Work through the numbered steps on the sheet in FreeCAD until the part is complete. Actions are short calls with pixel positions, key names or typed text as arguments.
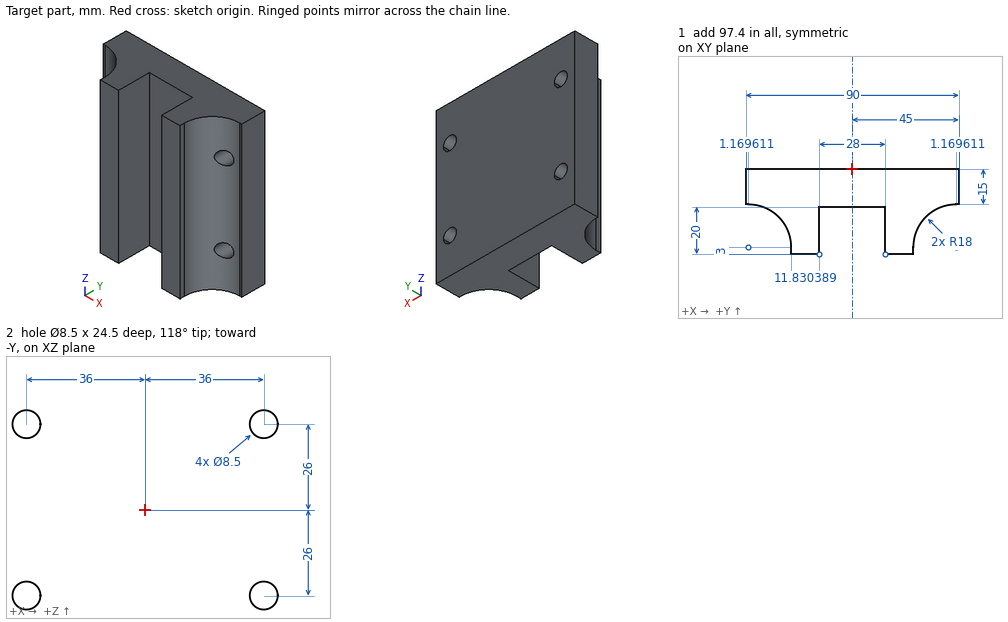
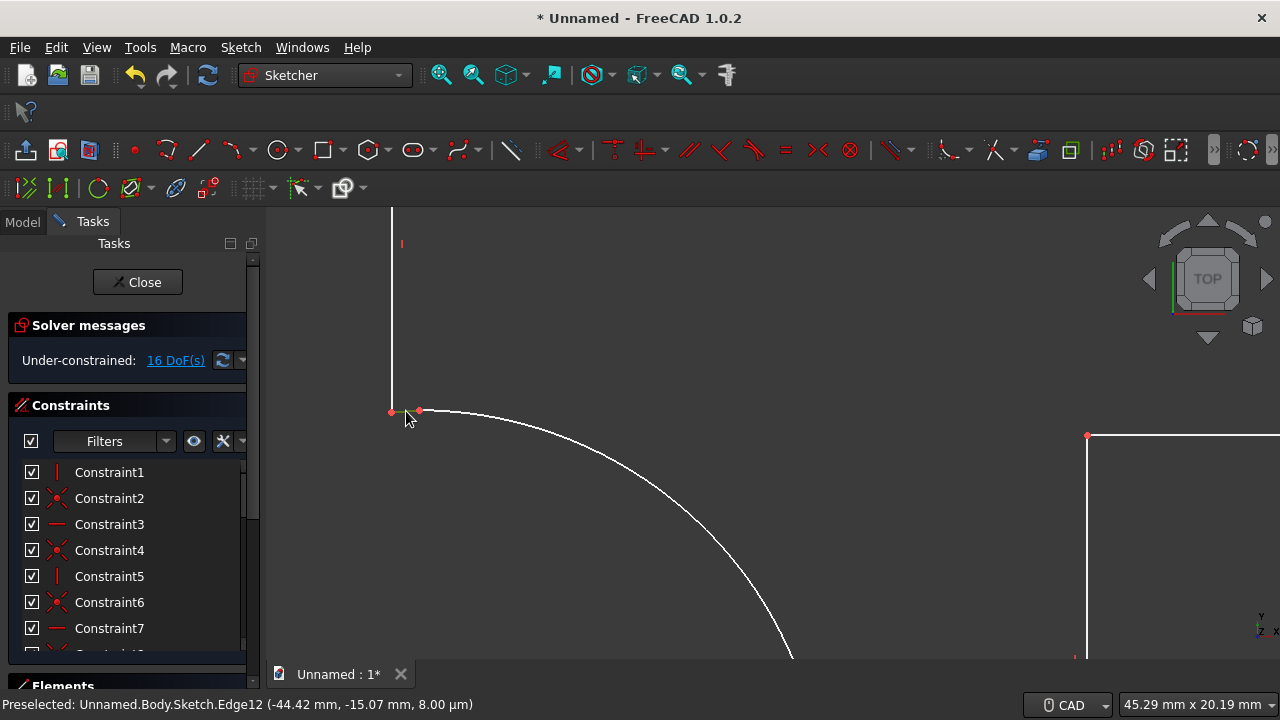
click(604, 455)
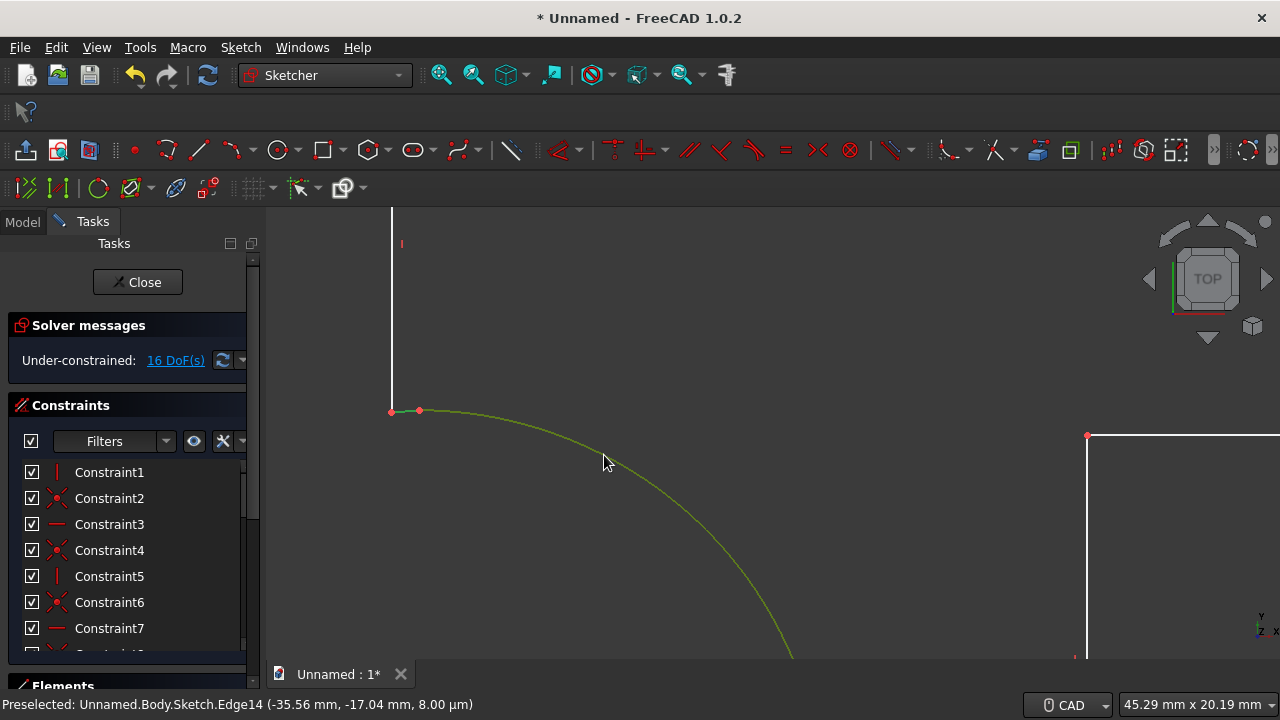
key(t)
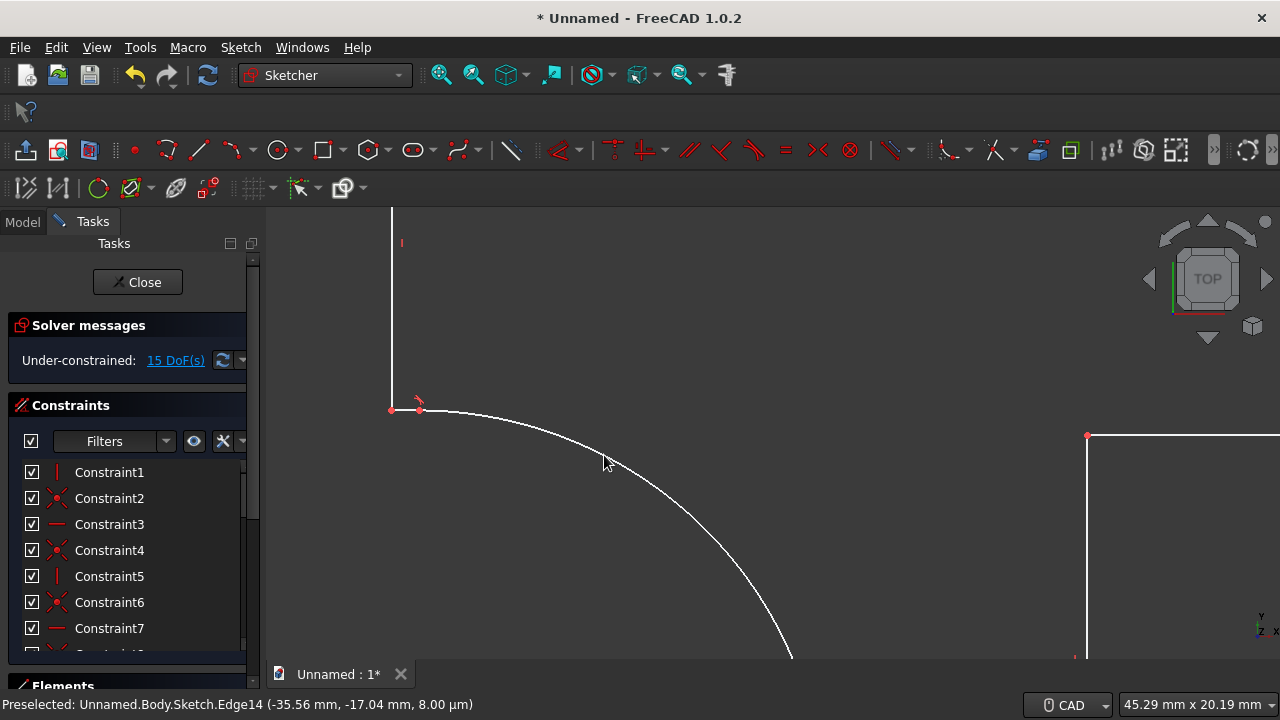
scroll(405, 414, down, 6)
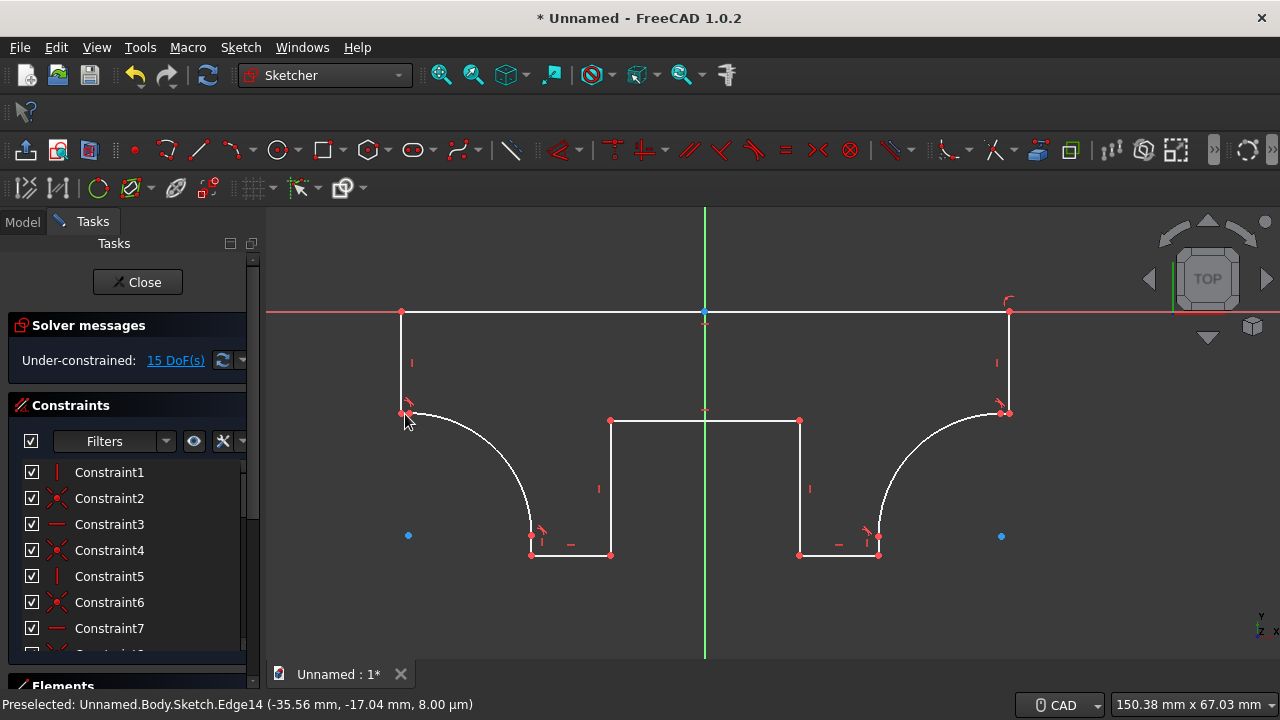
click(945, 427)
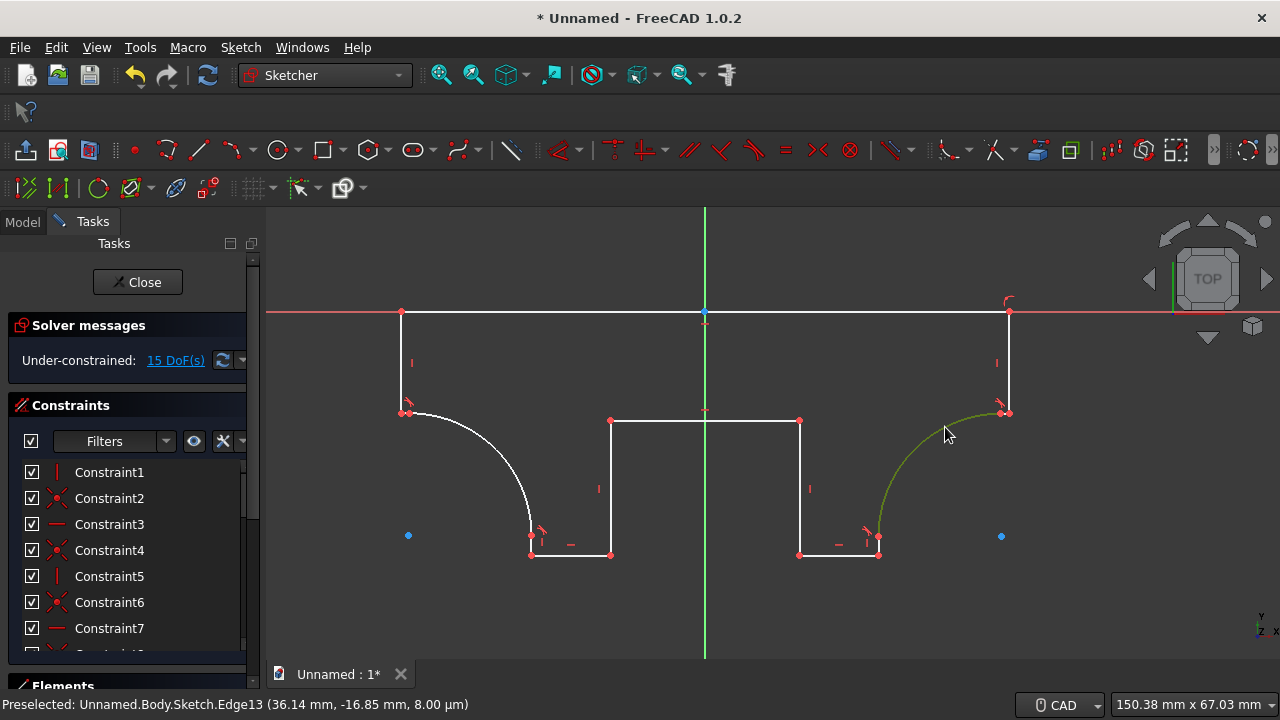
click(518, 480)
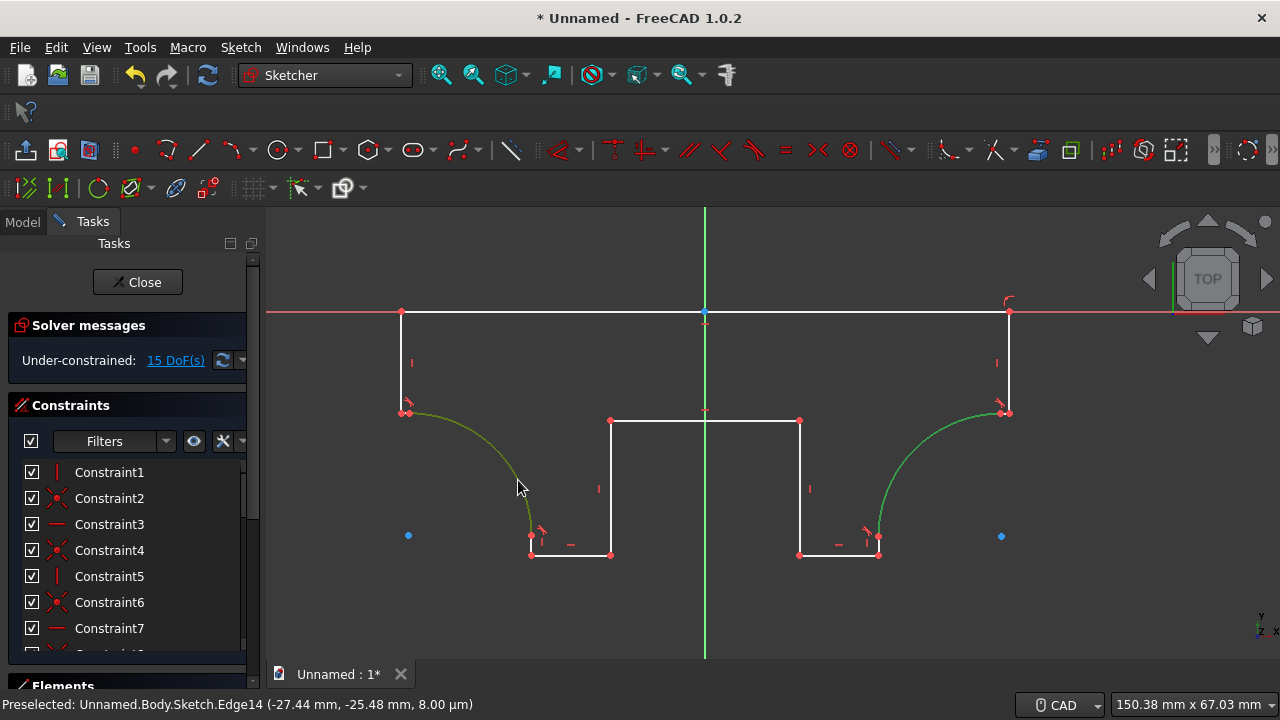
click(786, 150)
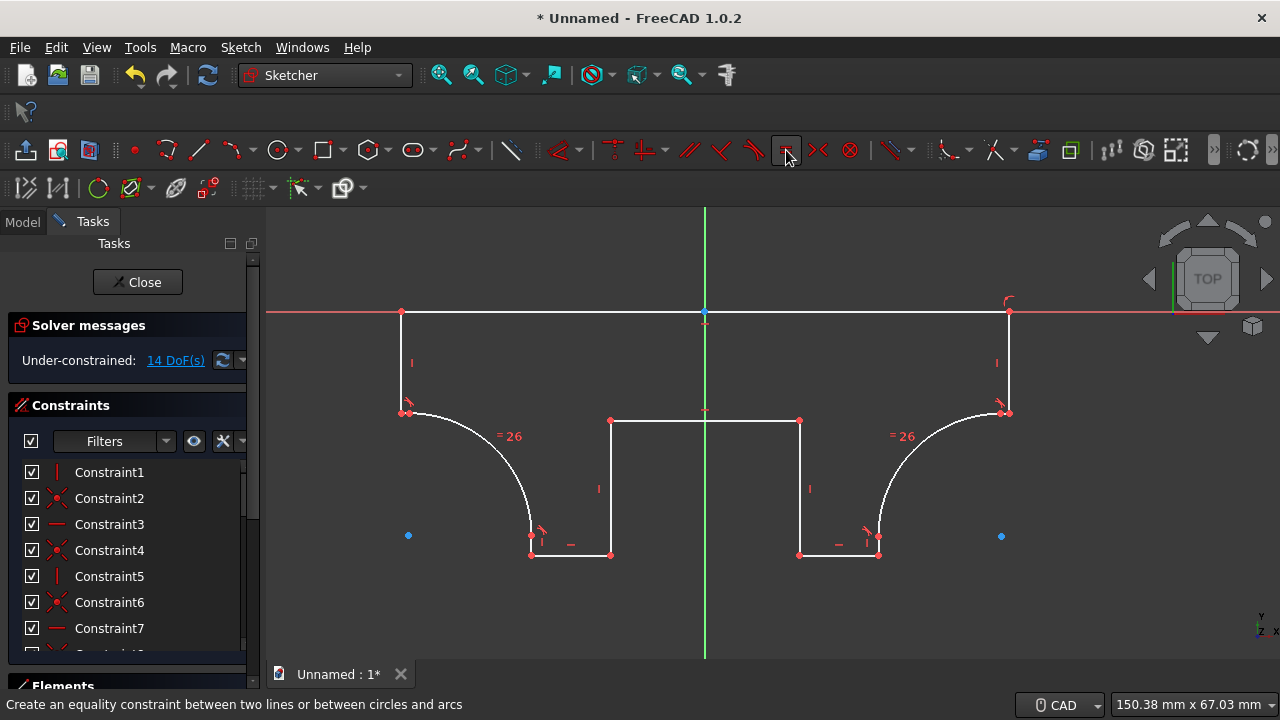
click(1001, 536)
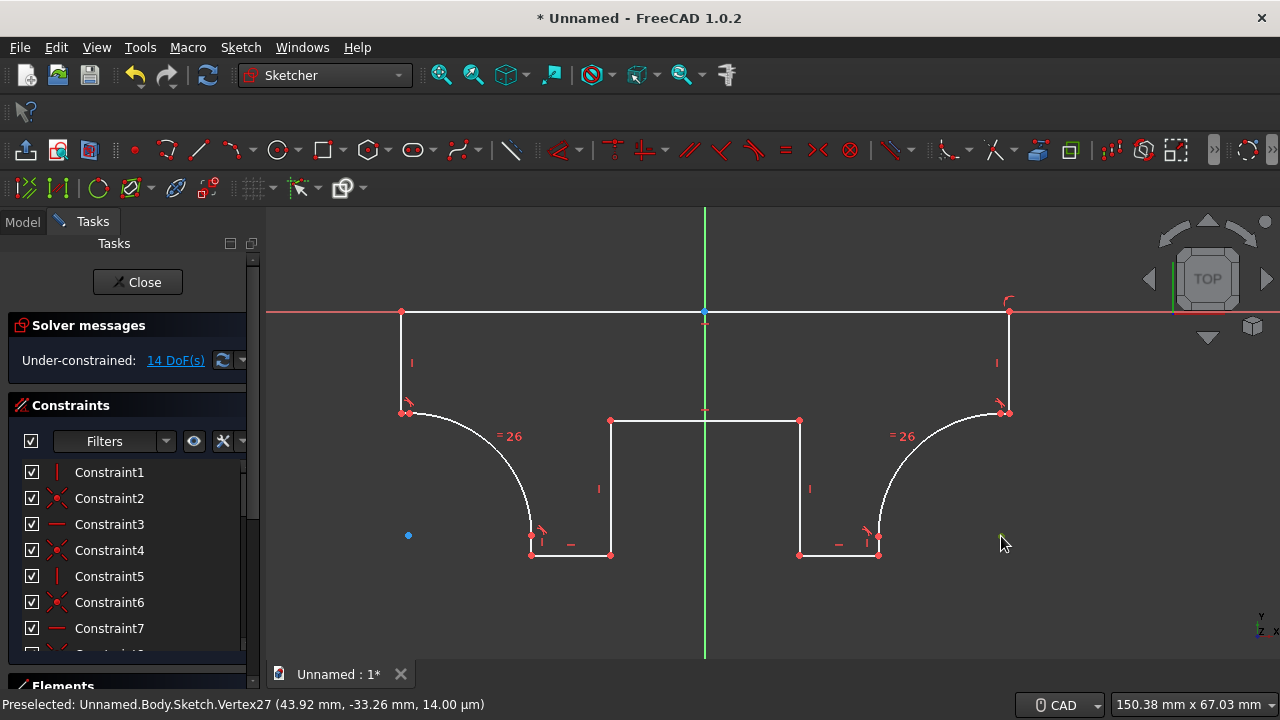
click(409, 536)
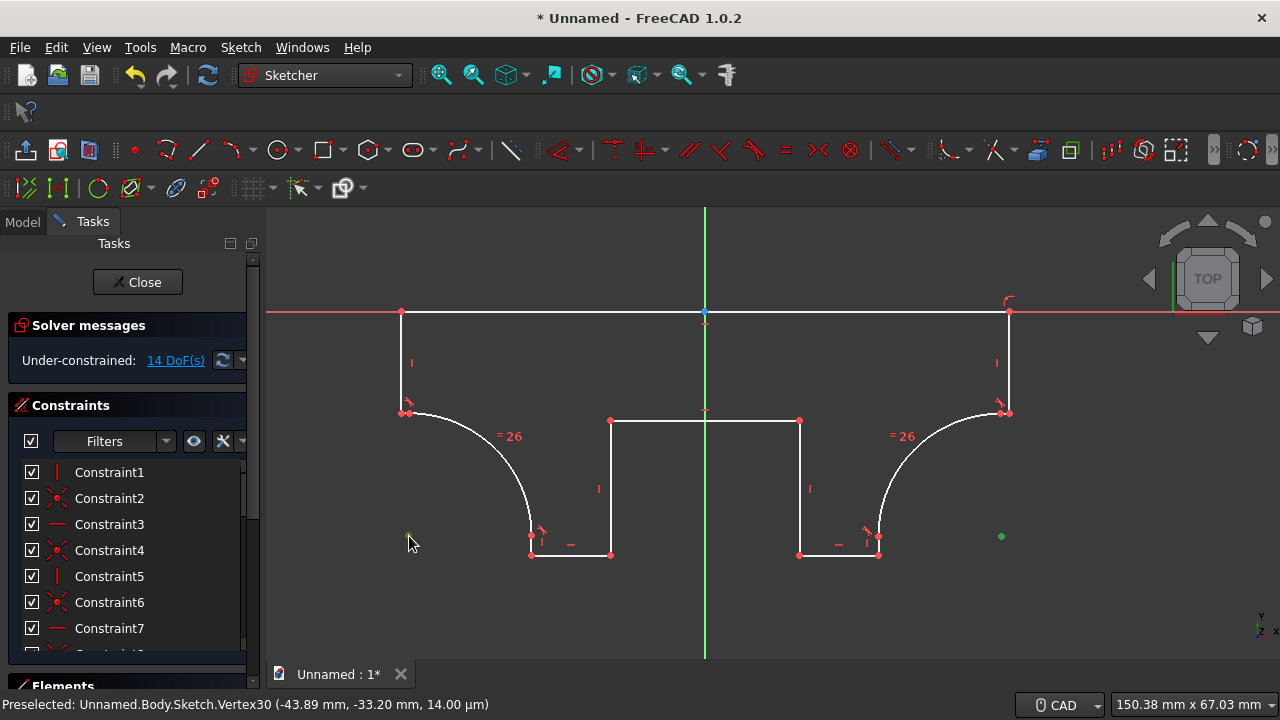
click(705, 603)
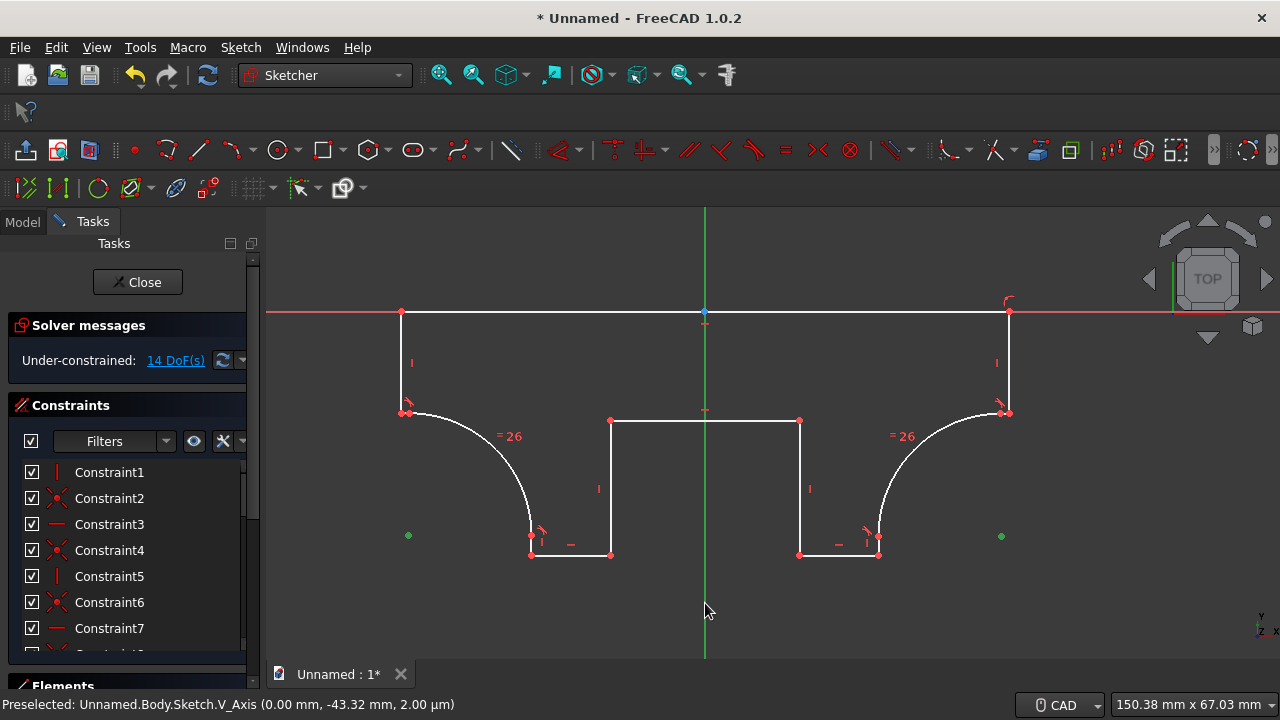
click(818, 150)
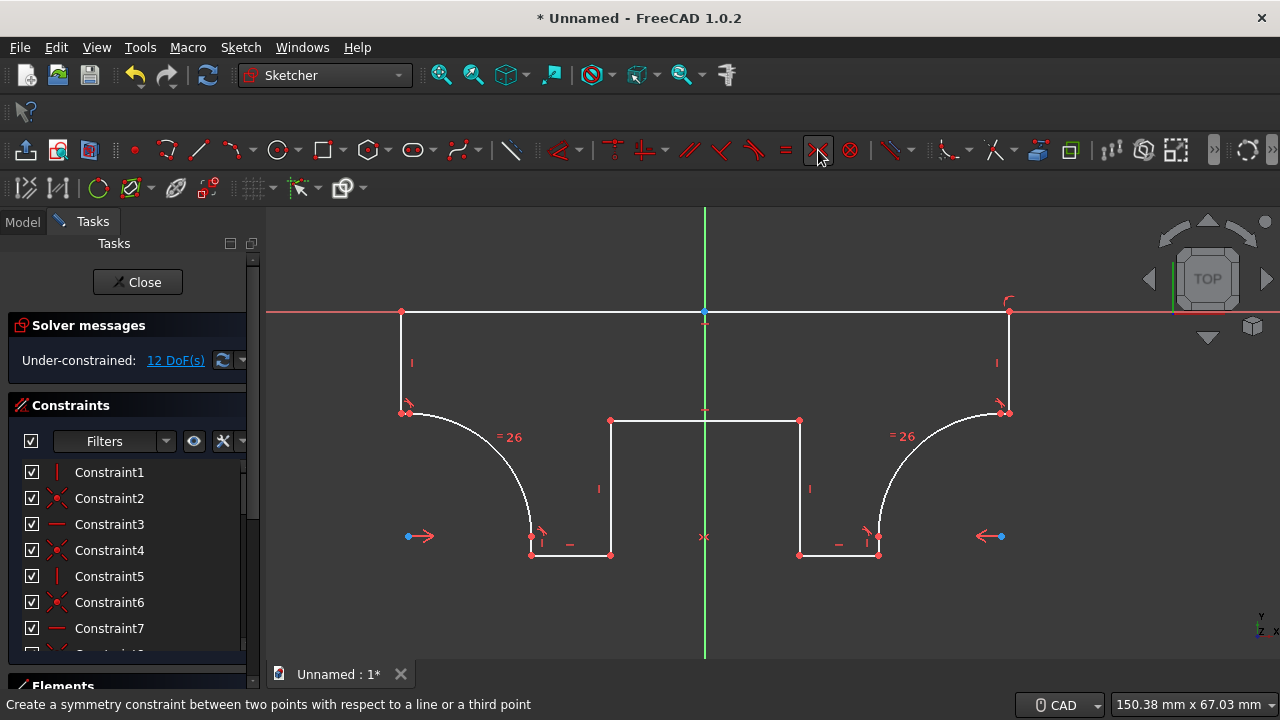
click(611, 556)